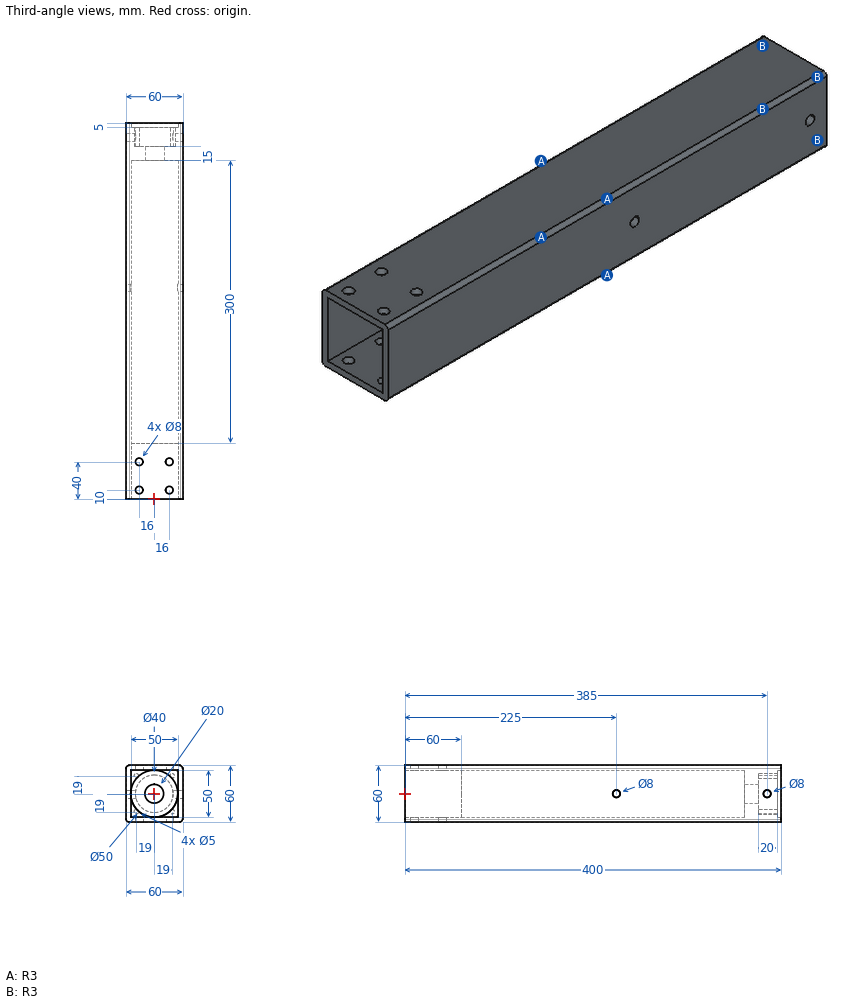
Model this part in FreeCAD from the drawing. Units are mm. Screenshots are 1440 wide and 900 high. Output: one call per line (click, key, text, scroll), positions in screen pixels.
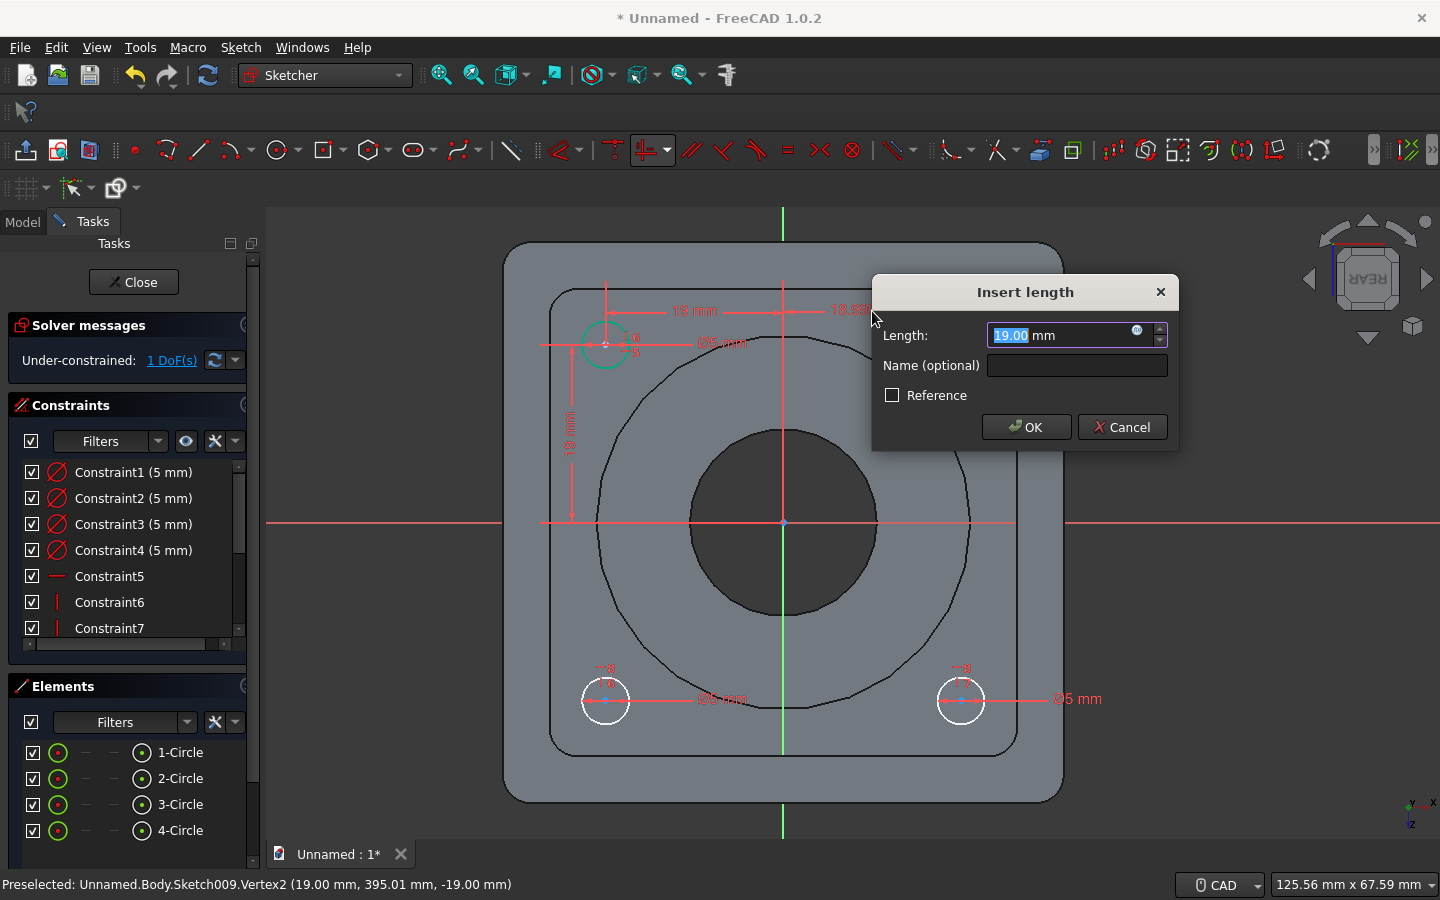
text(19)
key(Return)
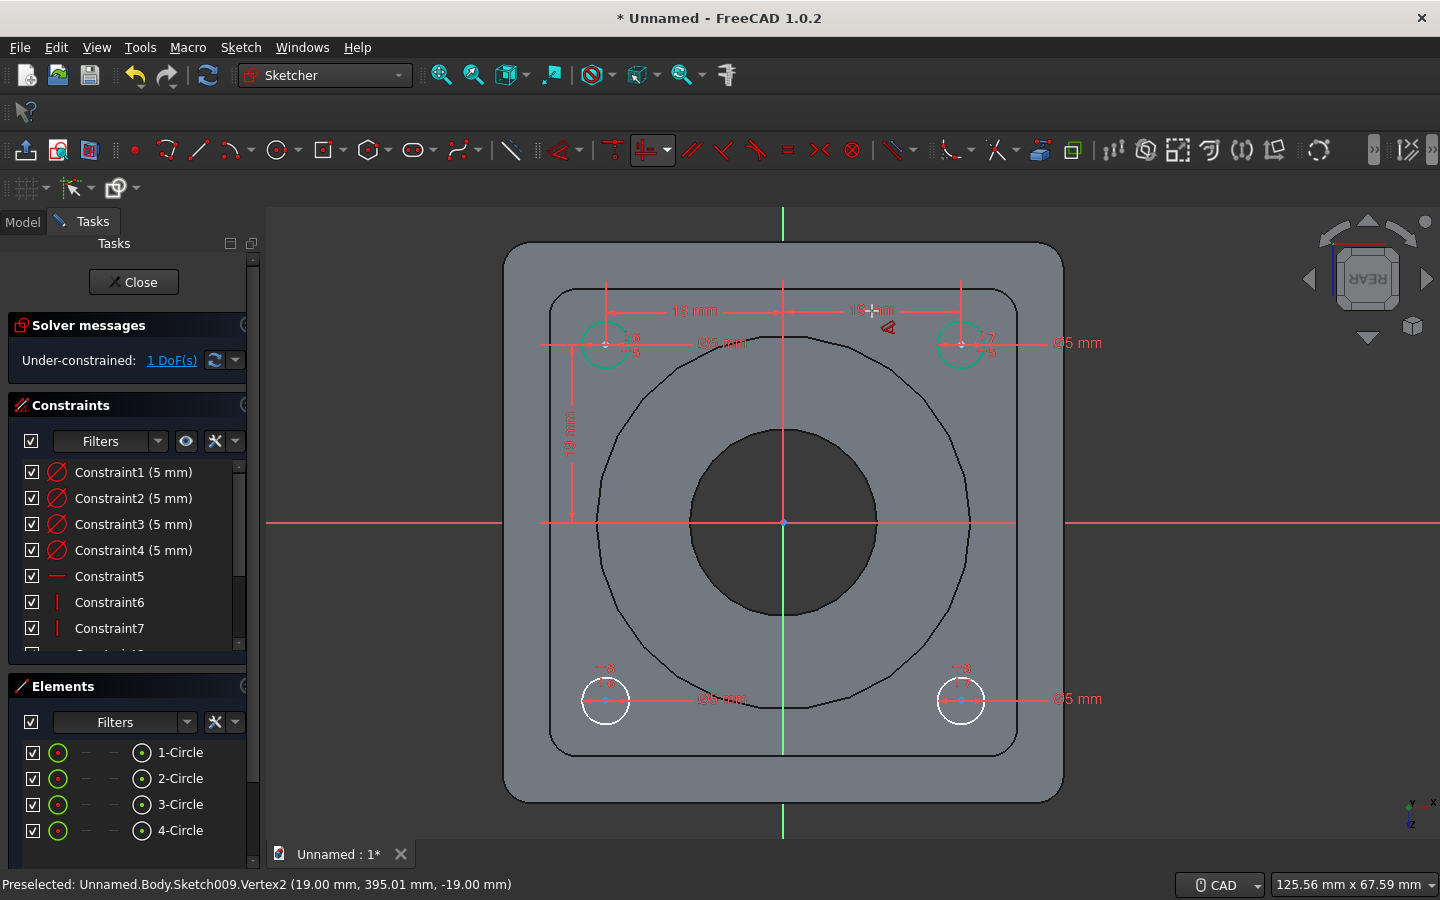
click(606, 701)
click(572, 612)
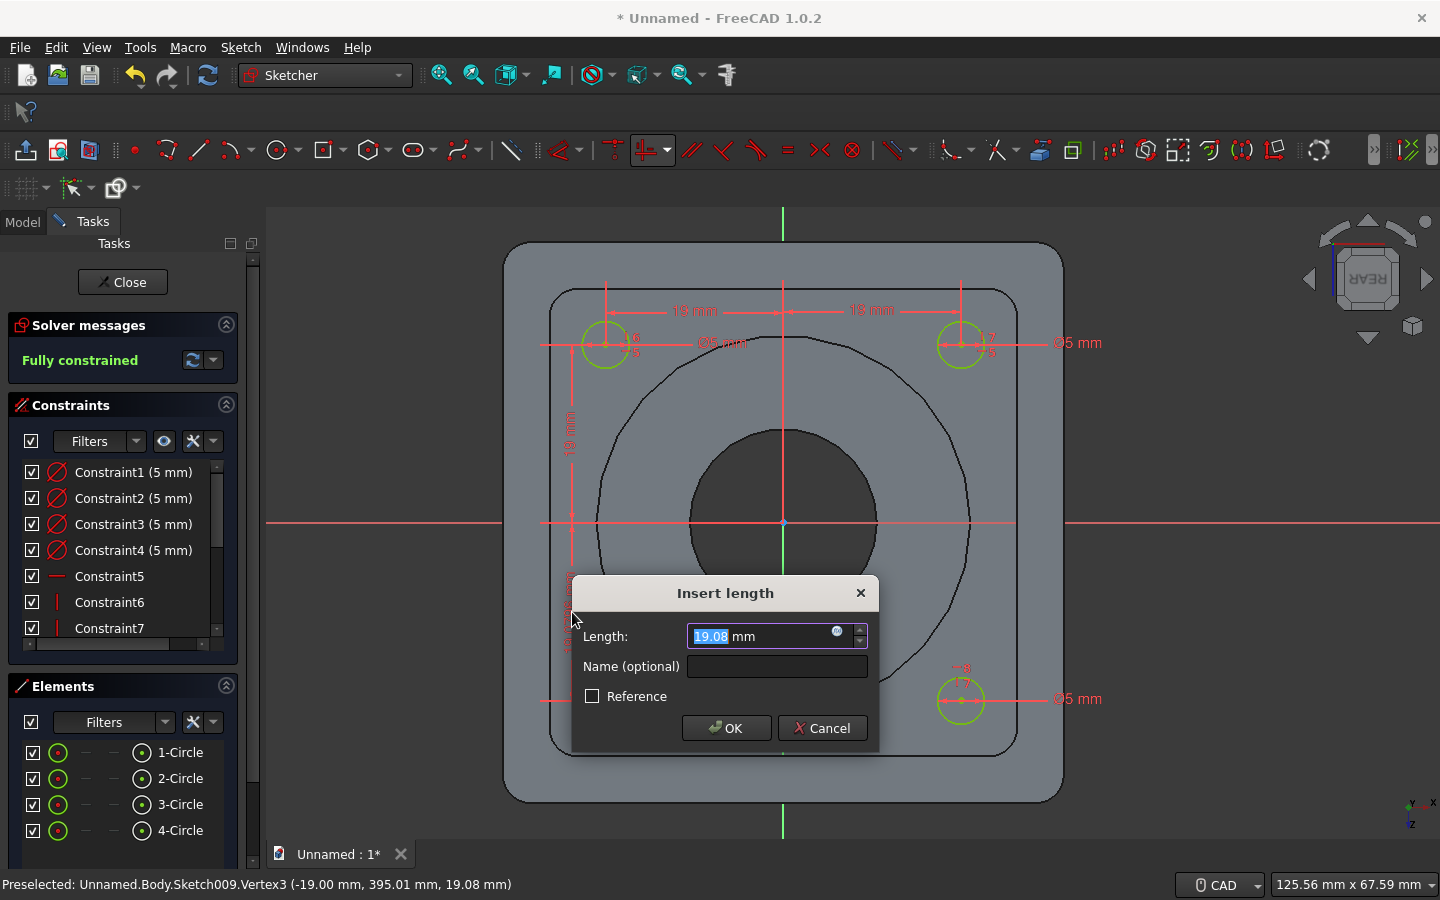
text(19)
key(Return)
key(Escape)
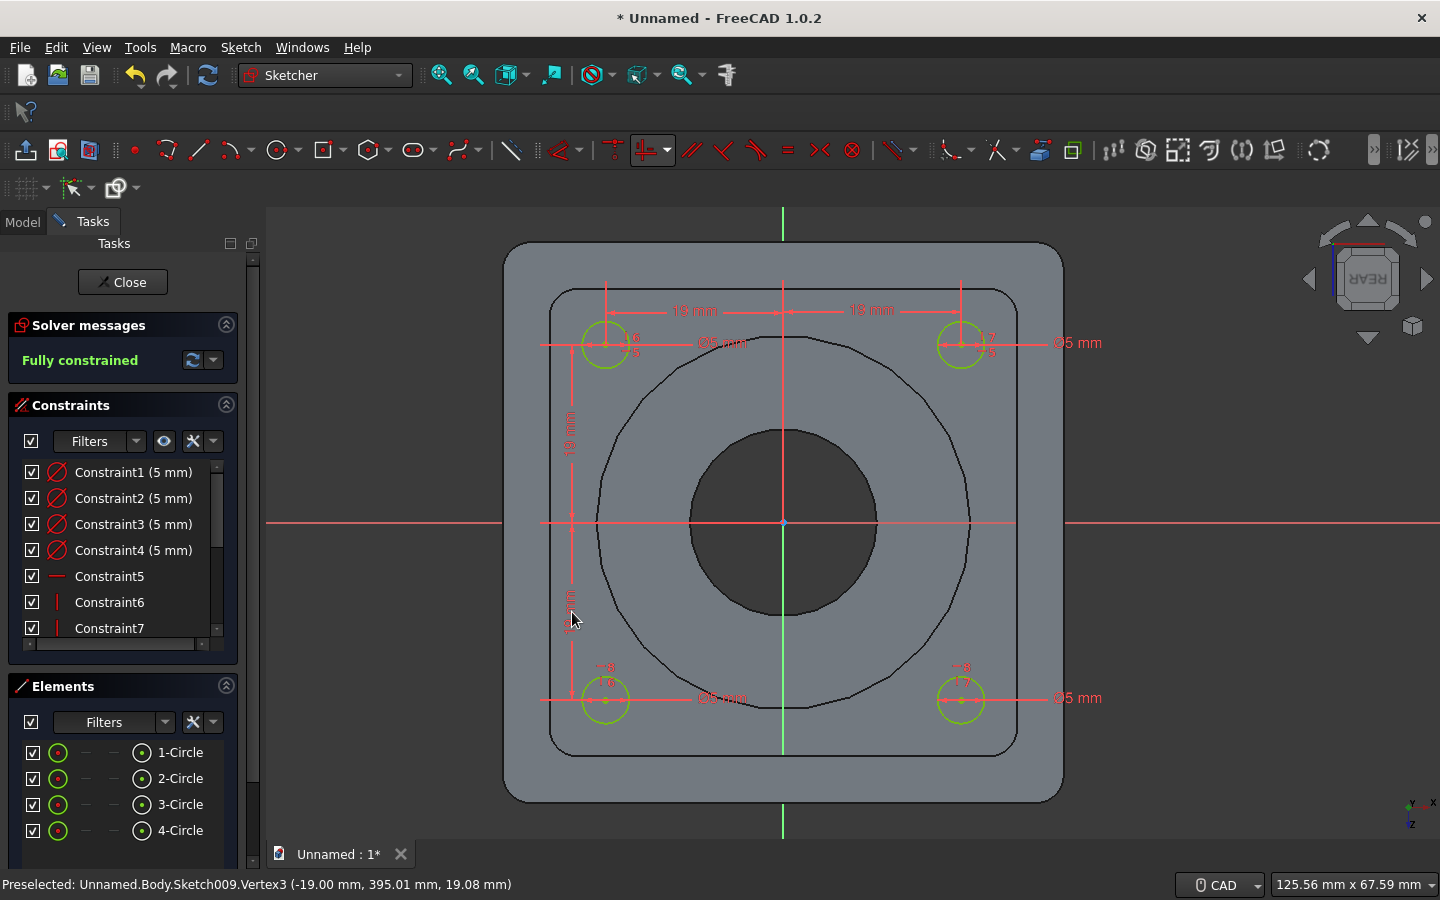
click(123, 282)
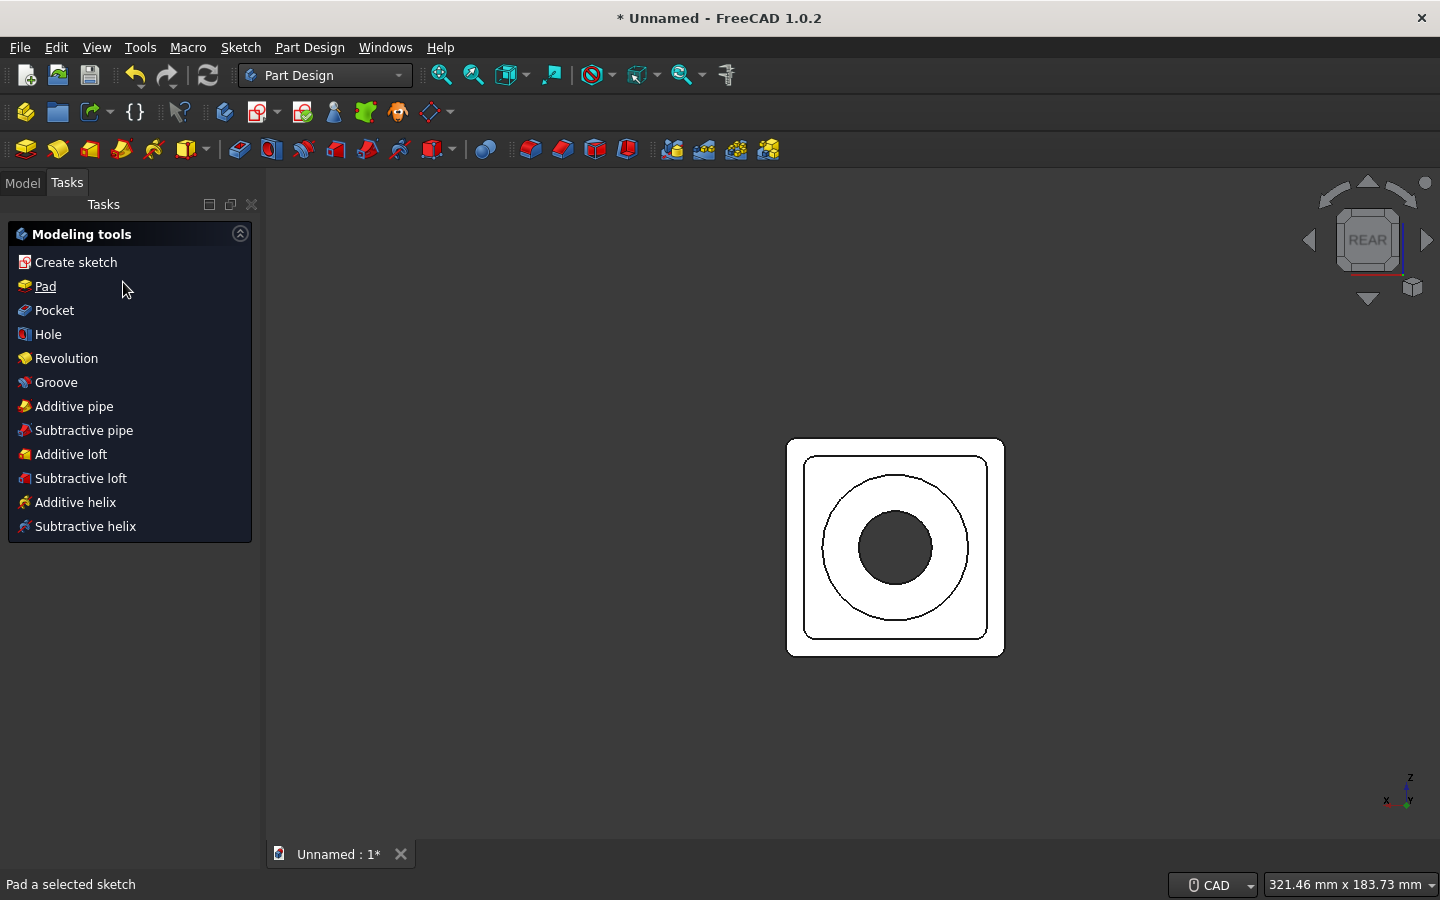
click(240, 150)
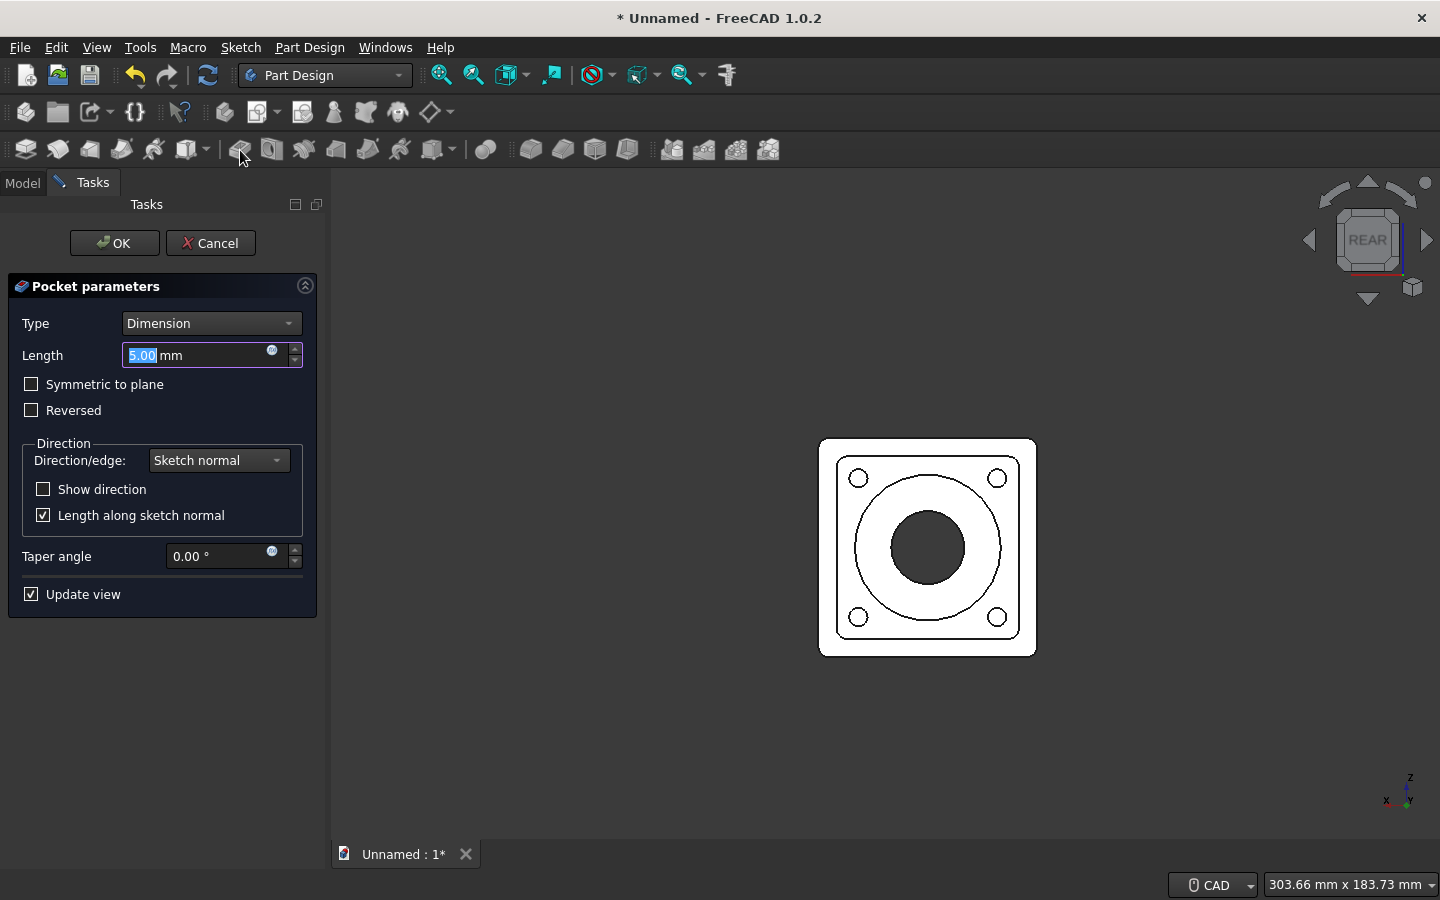
text(20)
key(Tab)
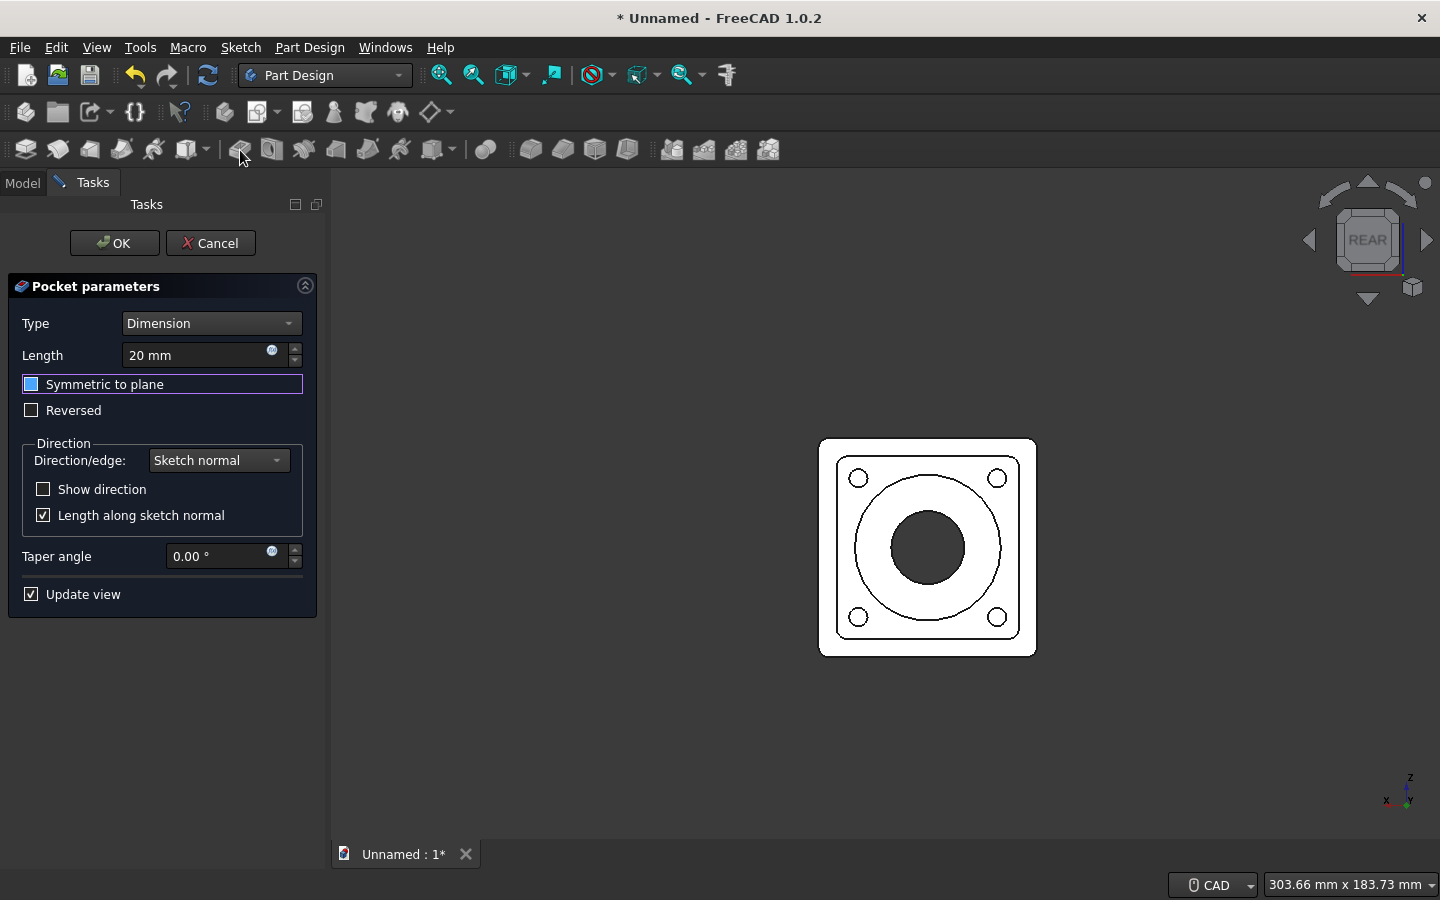
click(115, 243)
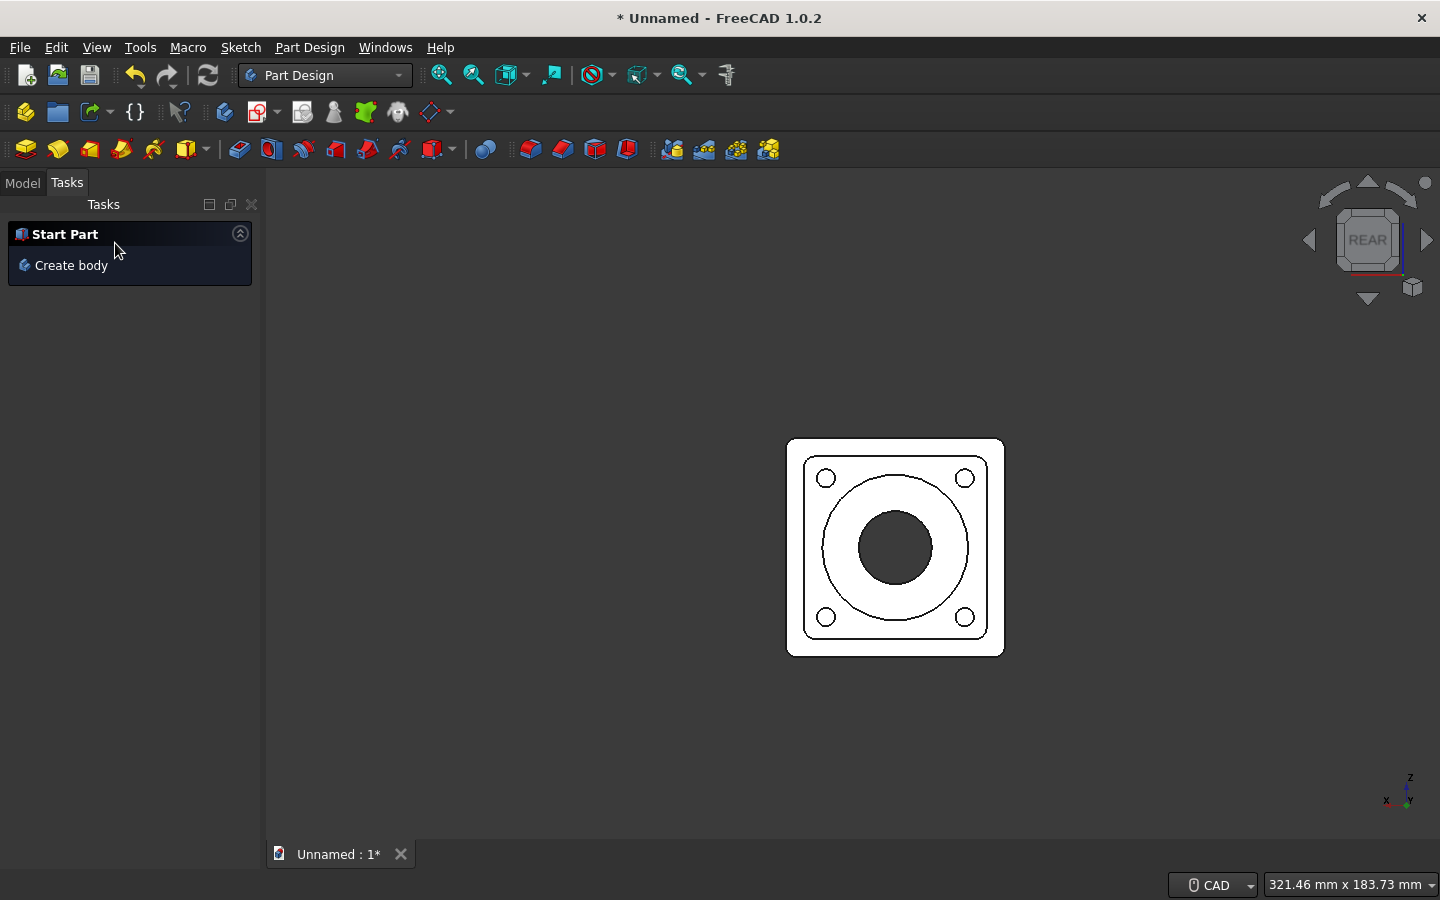
key(0)